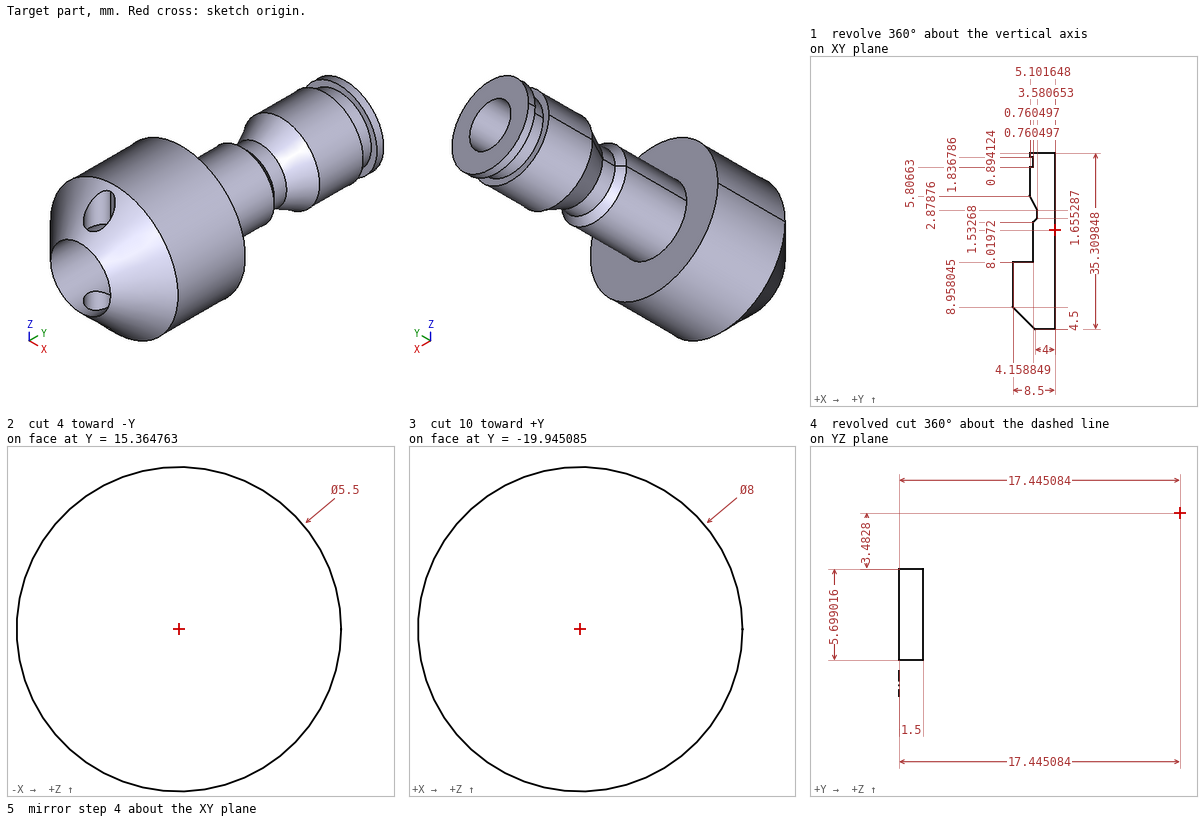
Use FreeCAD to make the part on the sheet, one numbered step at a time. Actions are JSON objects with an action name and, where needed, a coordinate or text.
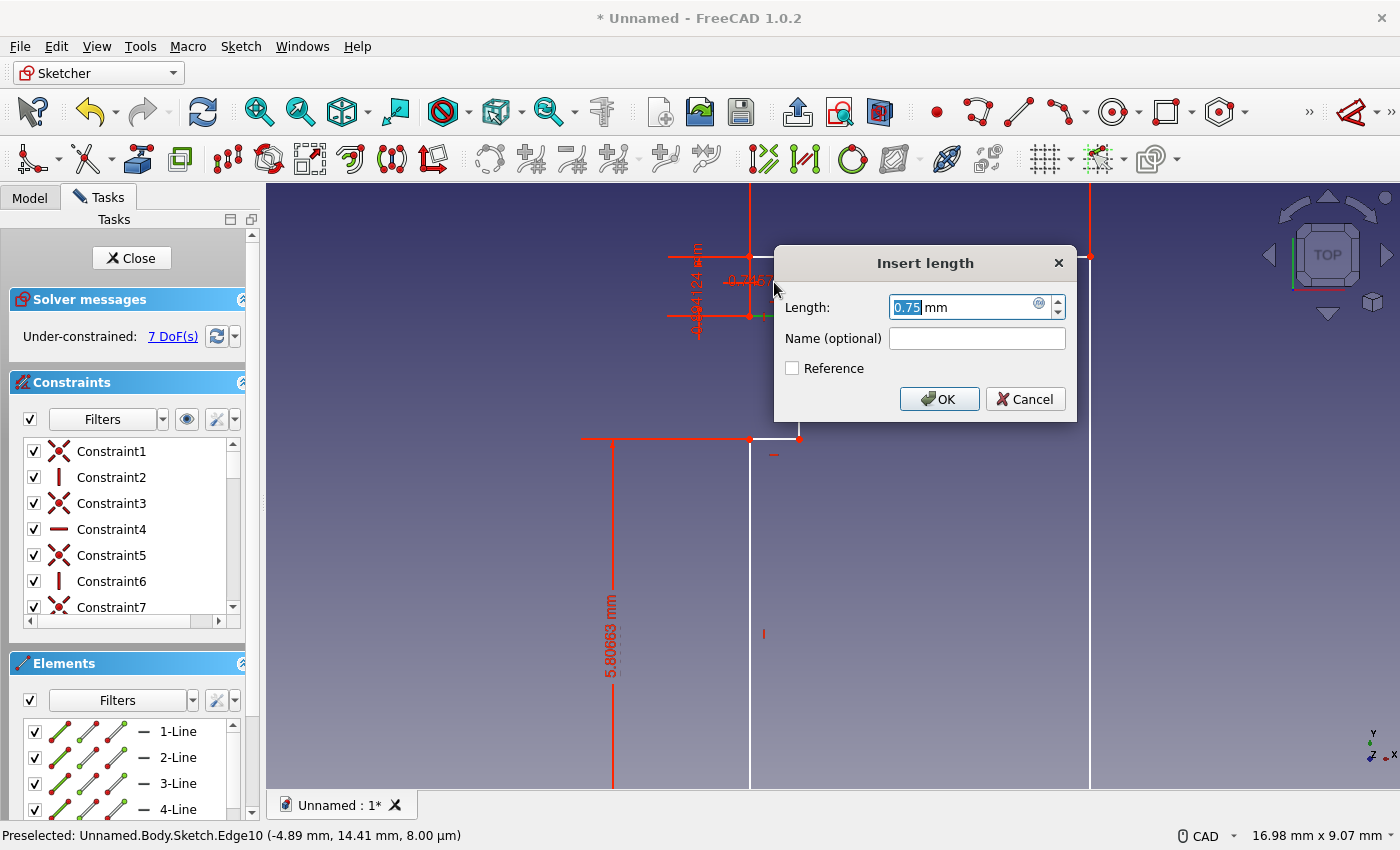
{"action": "type", "text": "0.760497"}
{"action": "key", "text": "Return"}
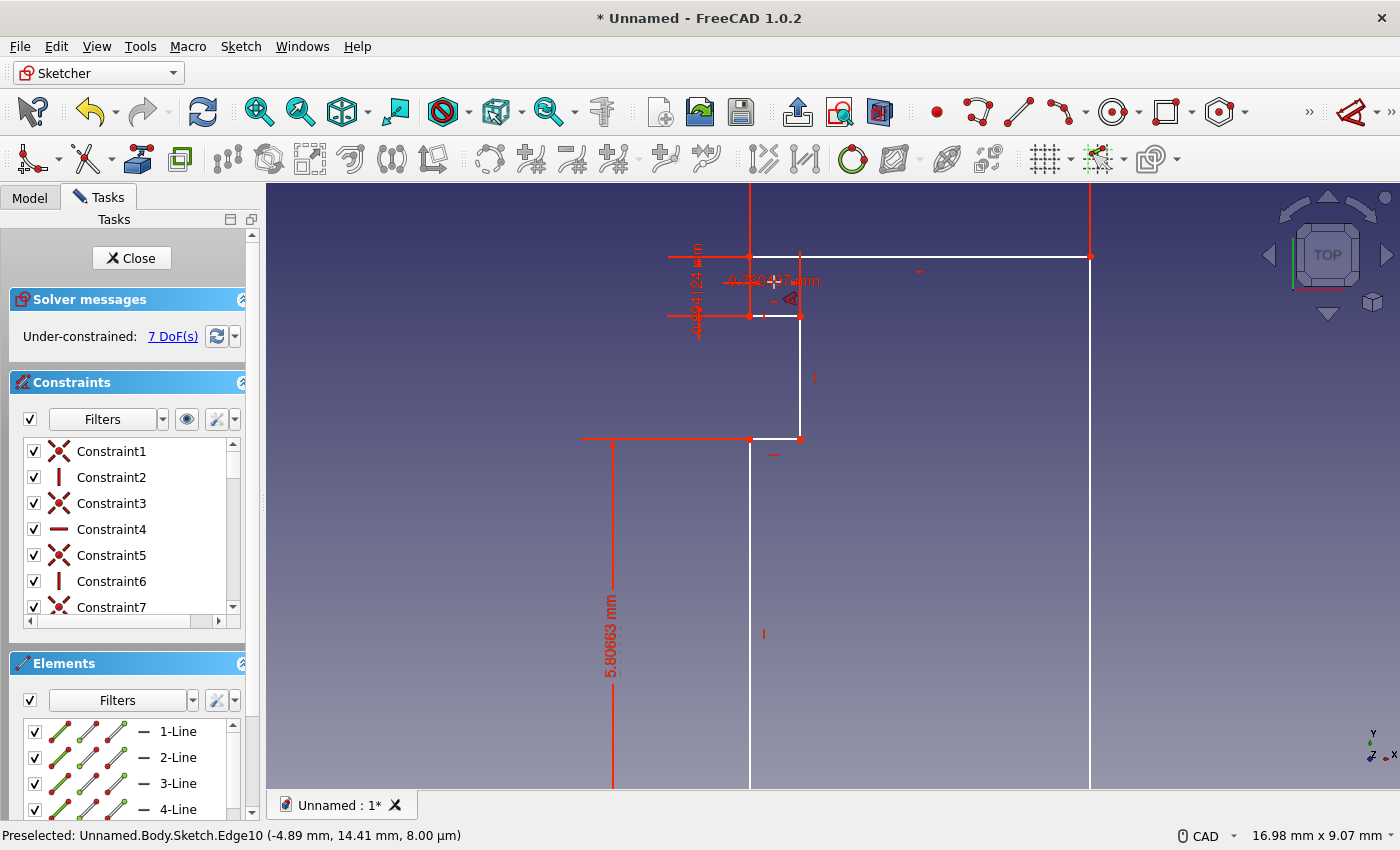
{"action": "left_click", "coordinate": [800, 353]}
{"action": "left_click", "coordinate": [766, 378]}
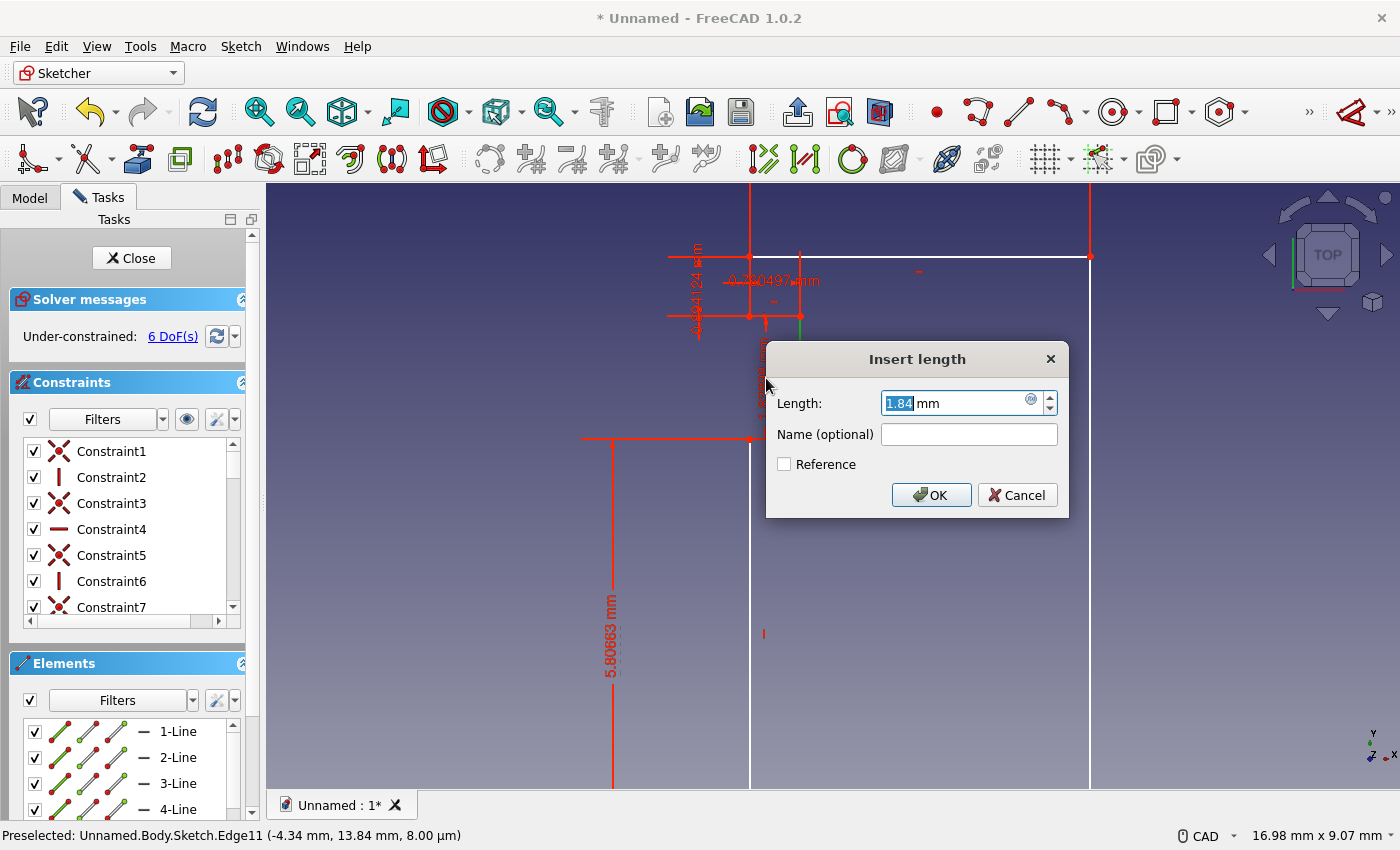
{"action": "type", "text": "1.836786"}
{"action": "key", "text": "Return"}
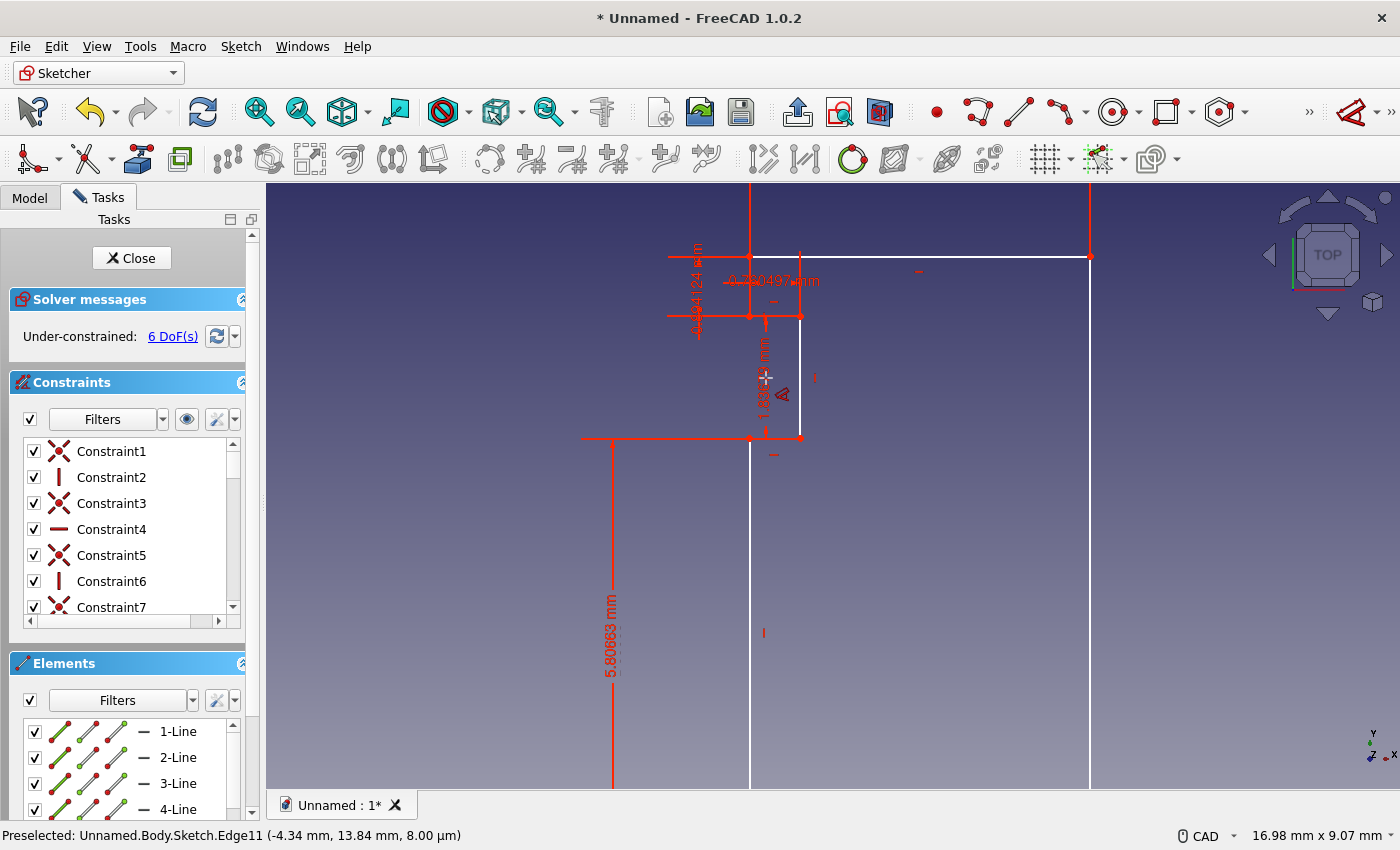
{"action": "left_click", "coordinate": [785, 439]}
{"action": "left_click", "coordinate": [775, 405]}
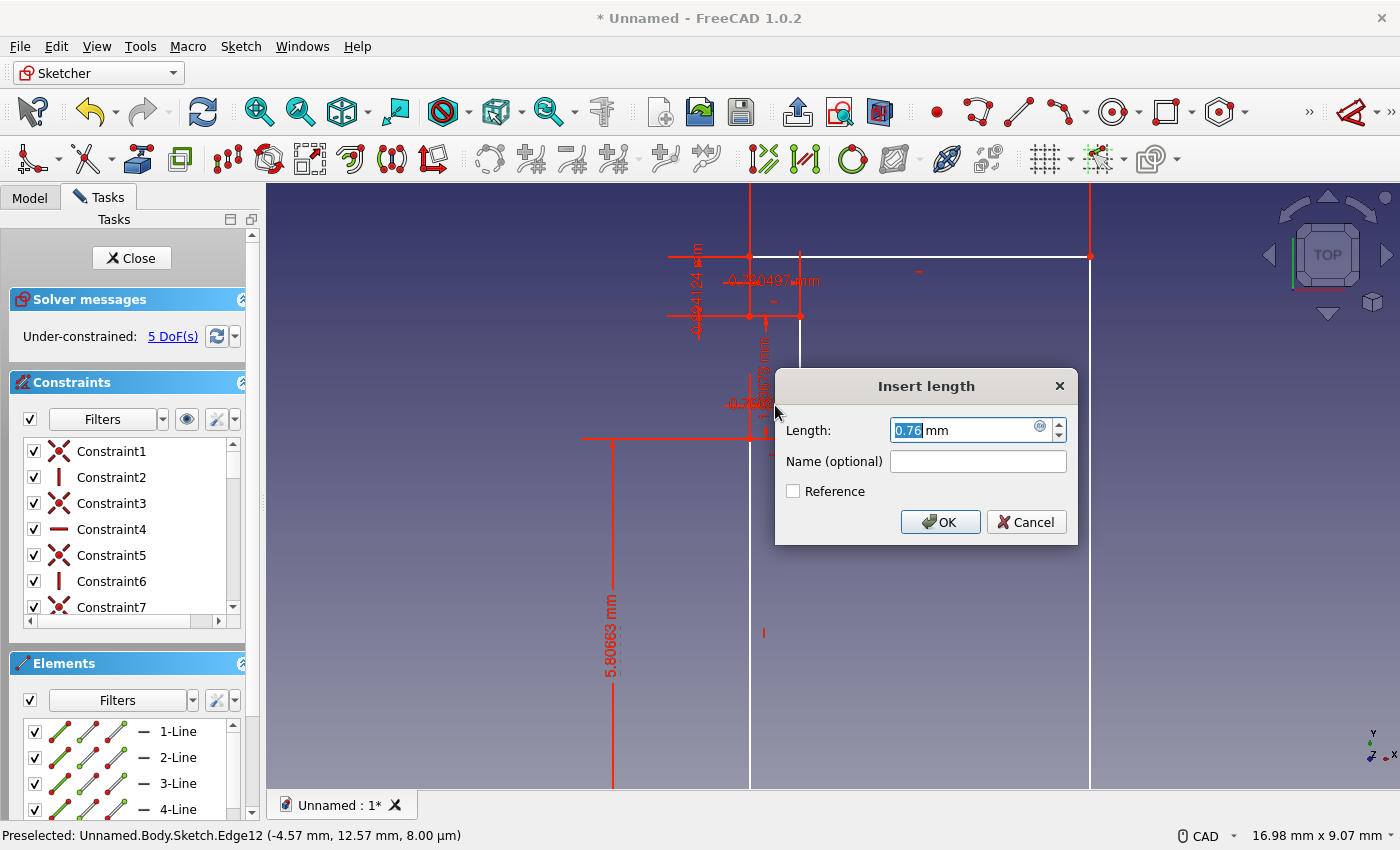
{"action": "type", "text": "0.760497"}
{"action": "key", "text": "Return"}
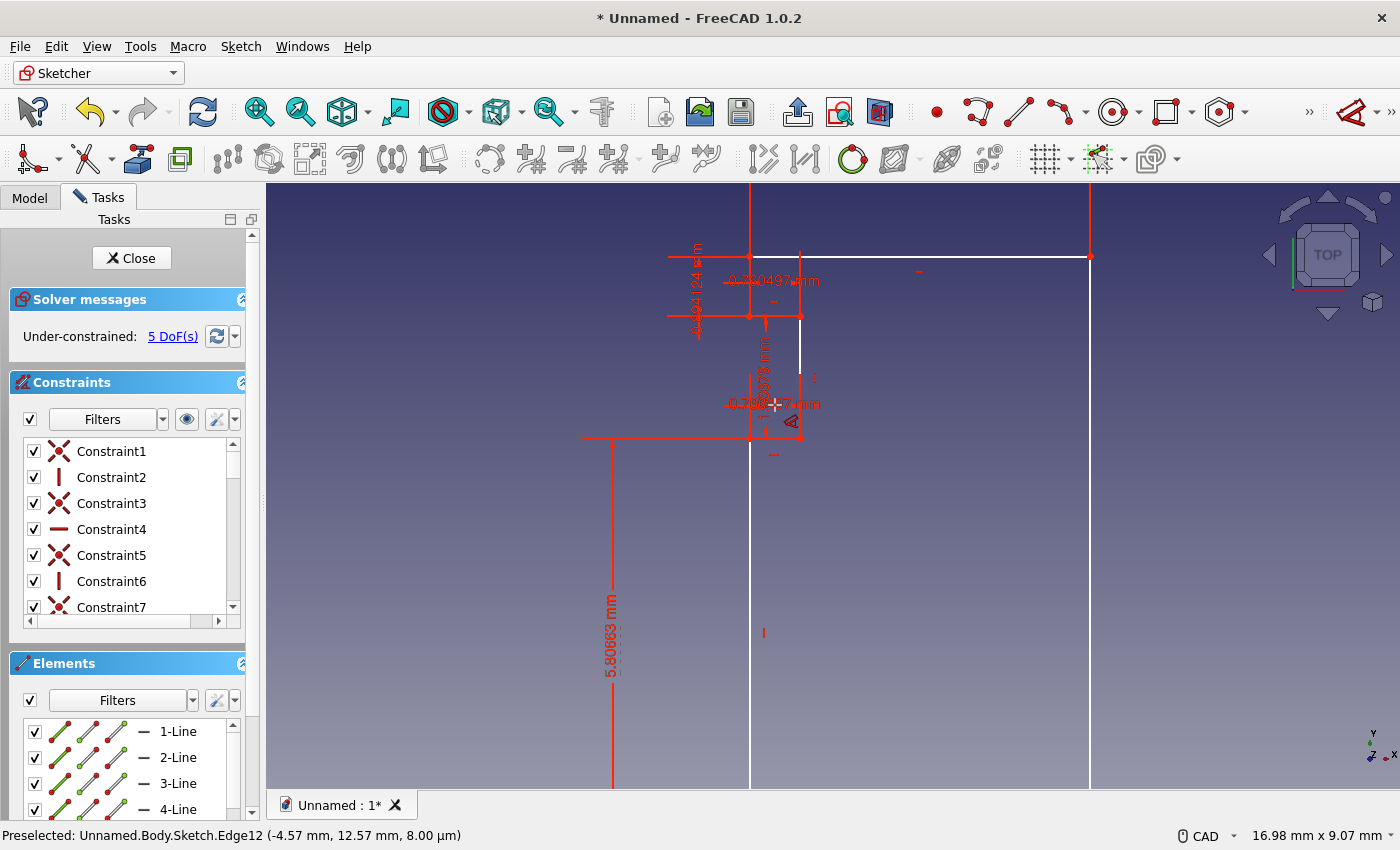
{"action": "scroll", "coordinate": [756, 299], "scroll_direction": "down", "scroll_amount": 9}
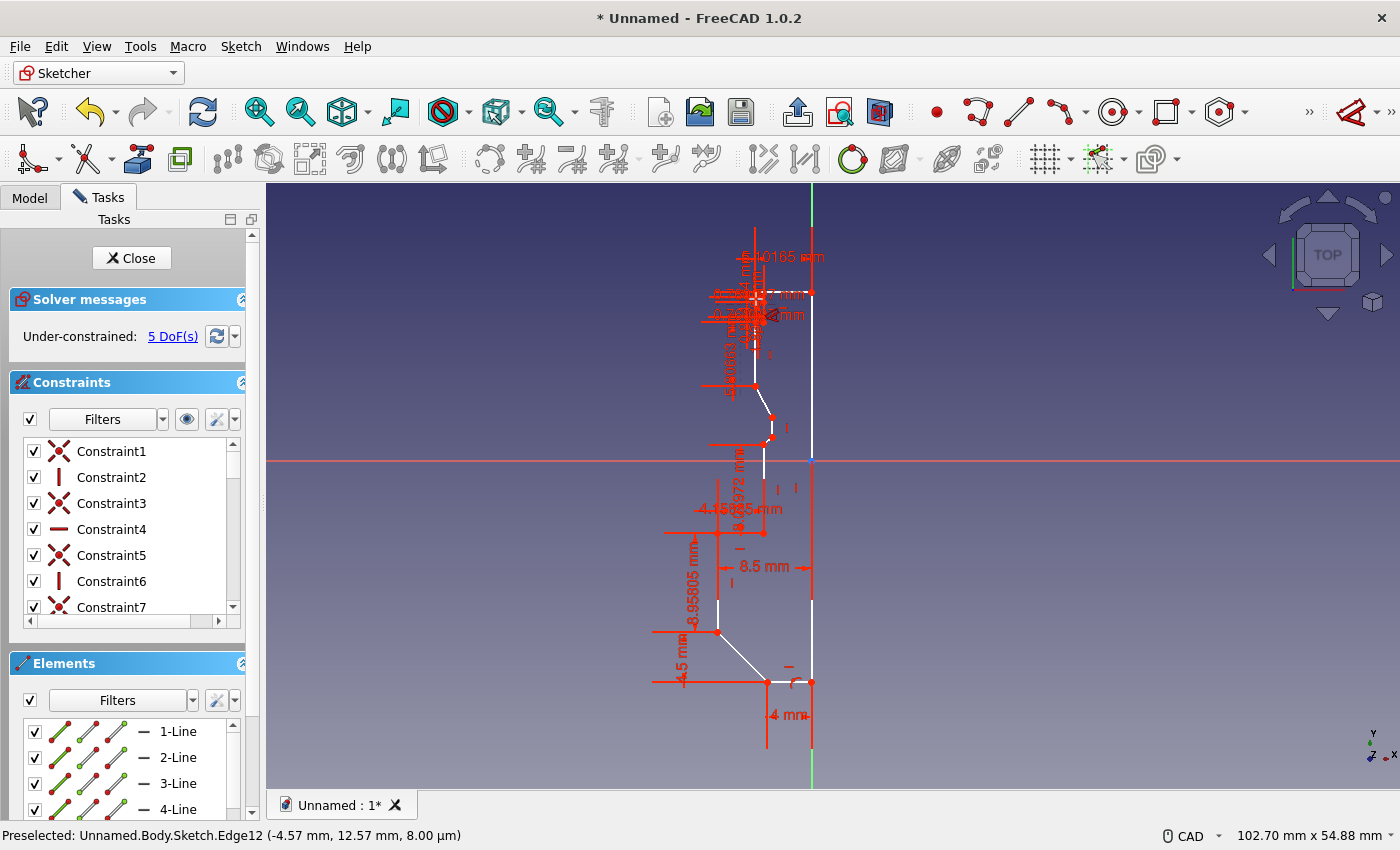
{"action": "scroll", "coordinate": [772, 424], "scroll_direction": "up", "scroll_amount": 5}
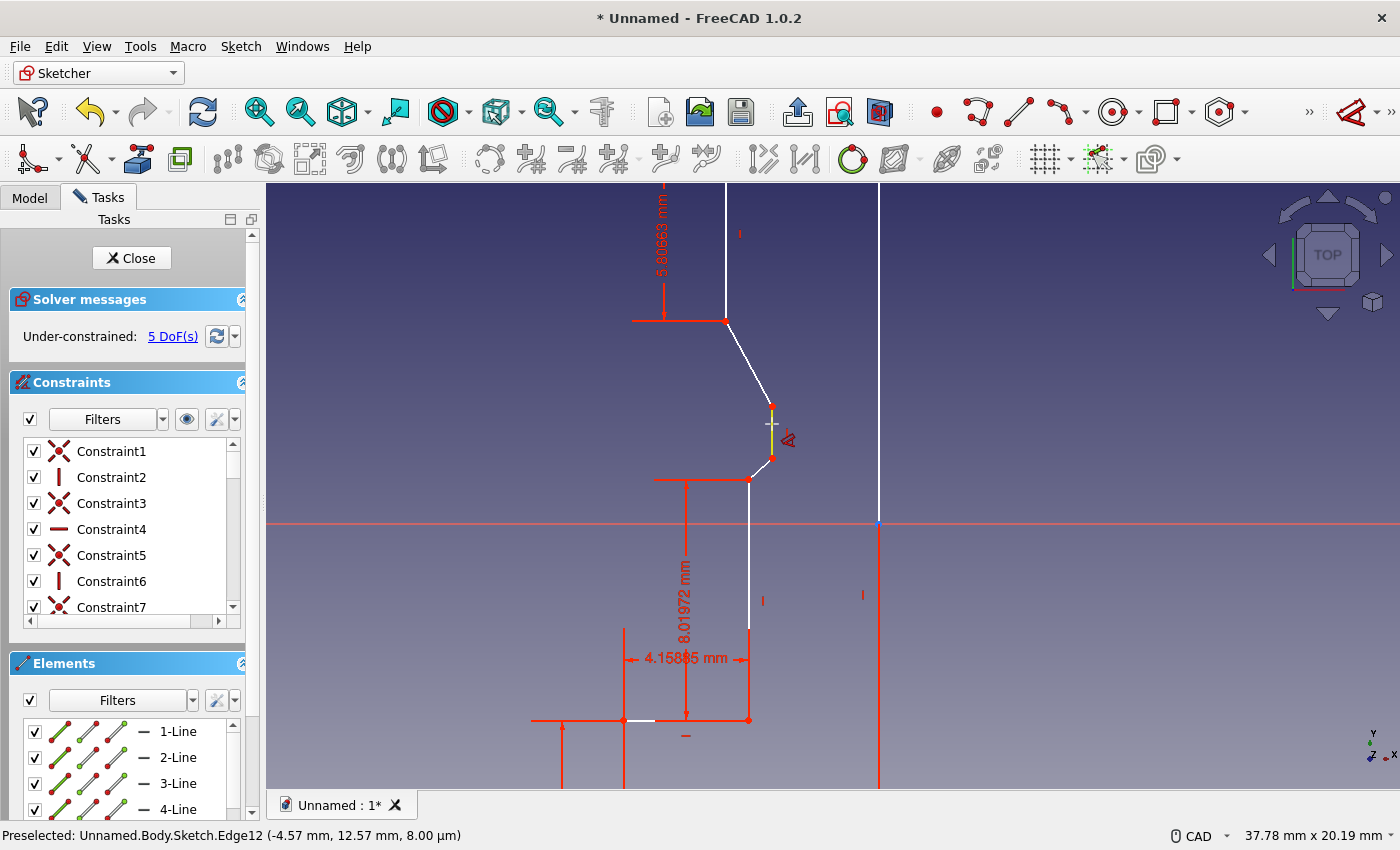
{"action": "left_click", "coordinate": [772, 422]}
{"action": "left_click", "coordinate": [806, 433]}